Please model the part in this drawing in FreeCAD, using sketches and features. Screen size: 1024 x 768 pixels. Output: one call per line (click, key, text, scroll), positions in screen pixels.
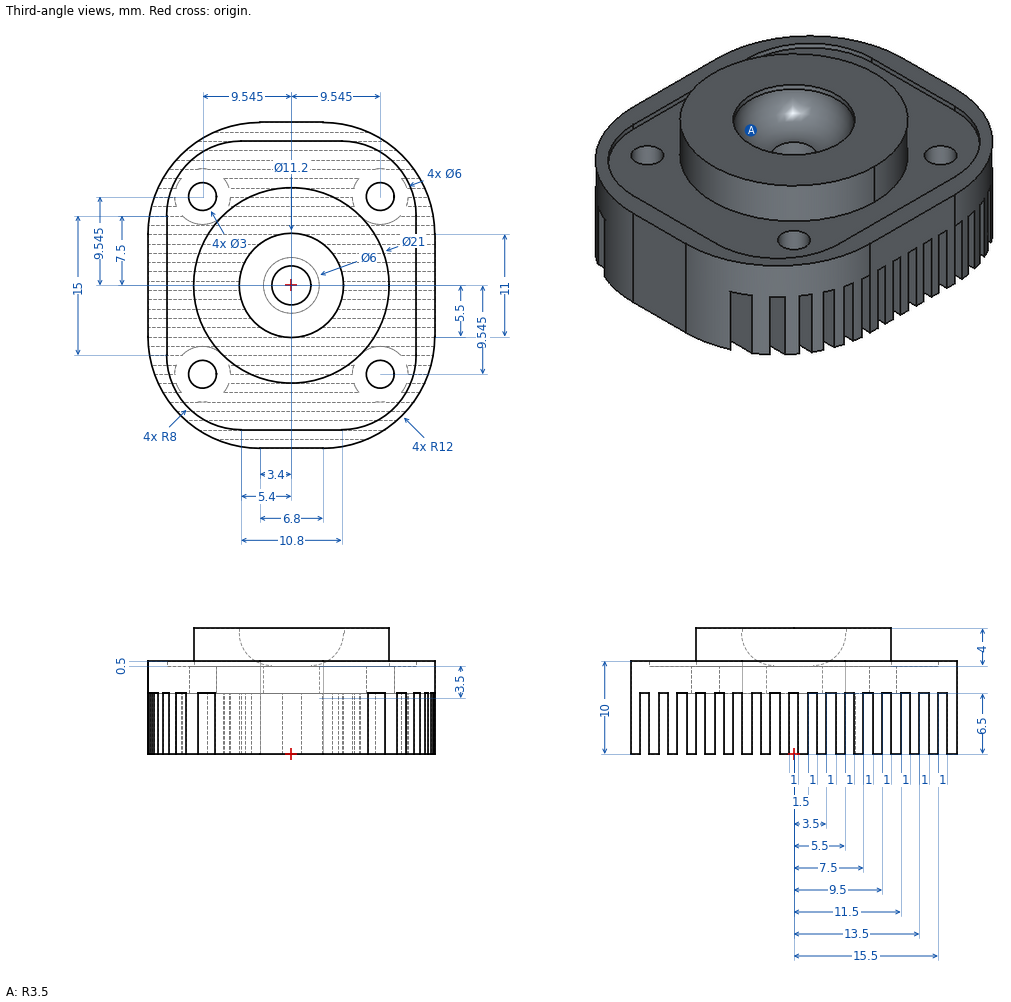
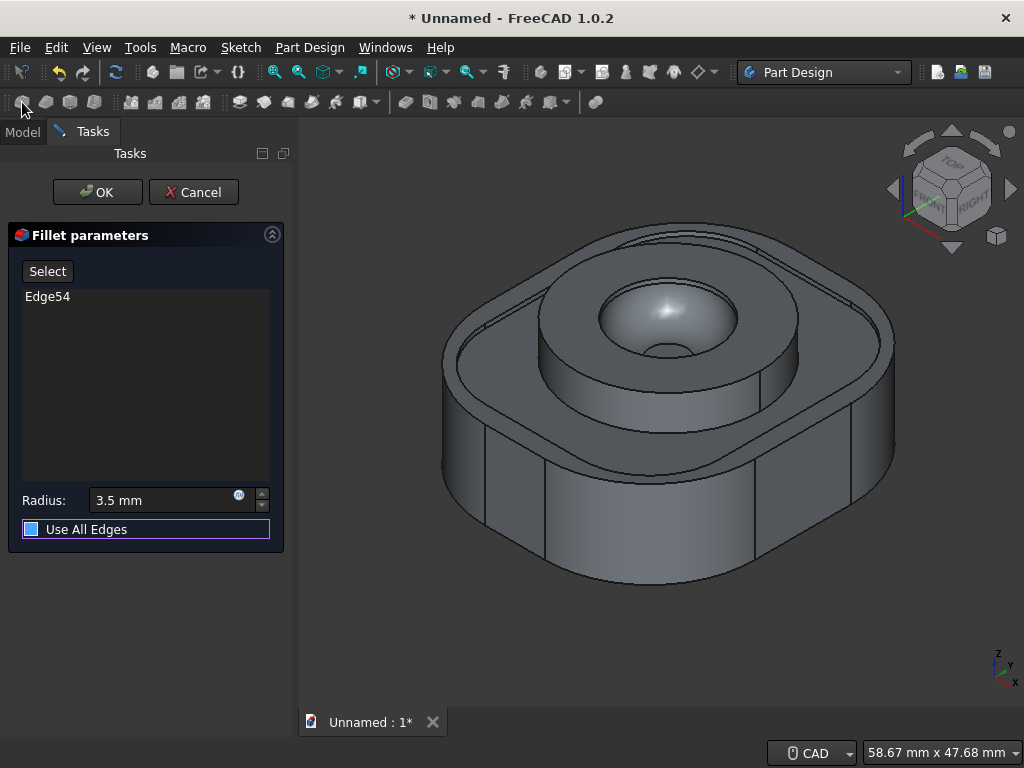
click(98, 192)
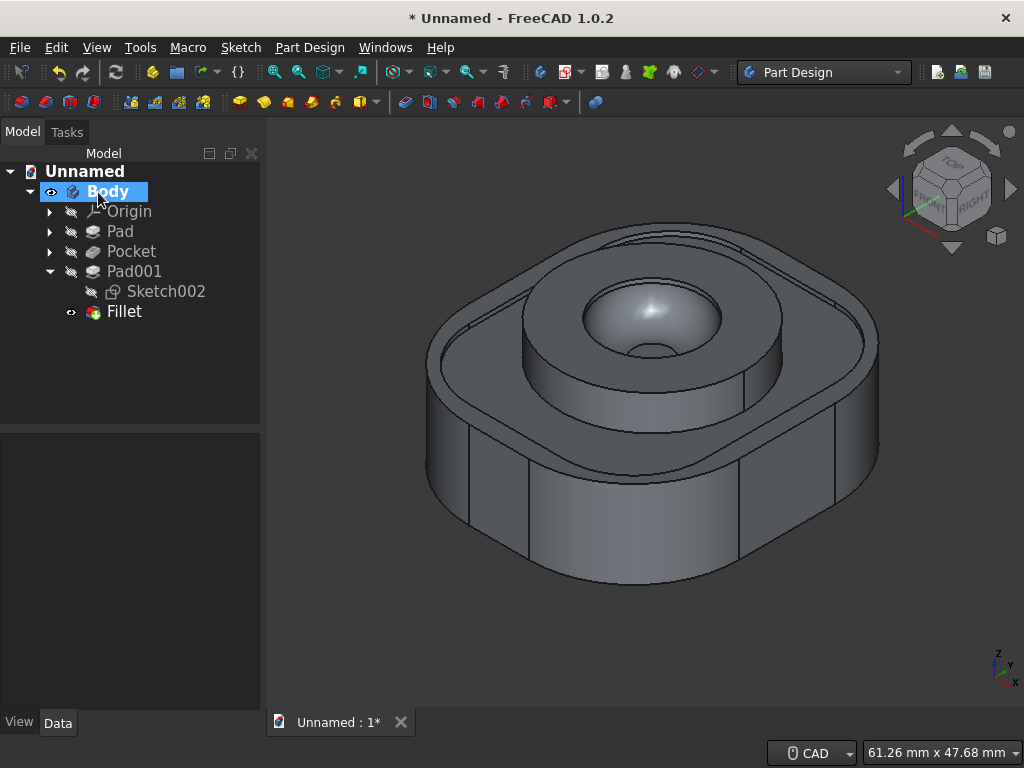
click(802, 310)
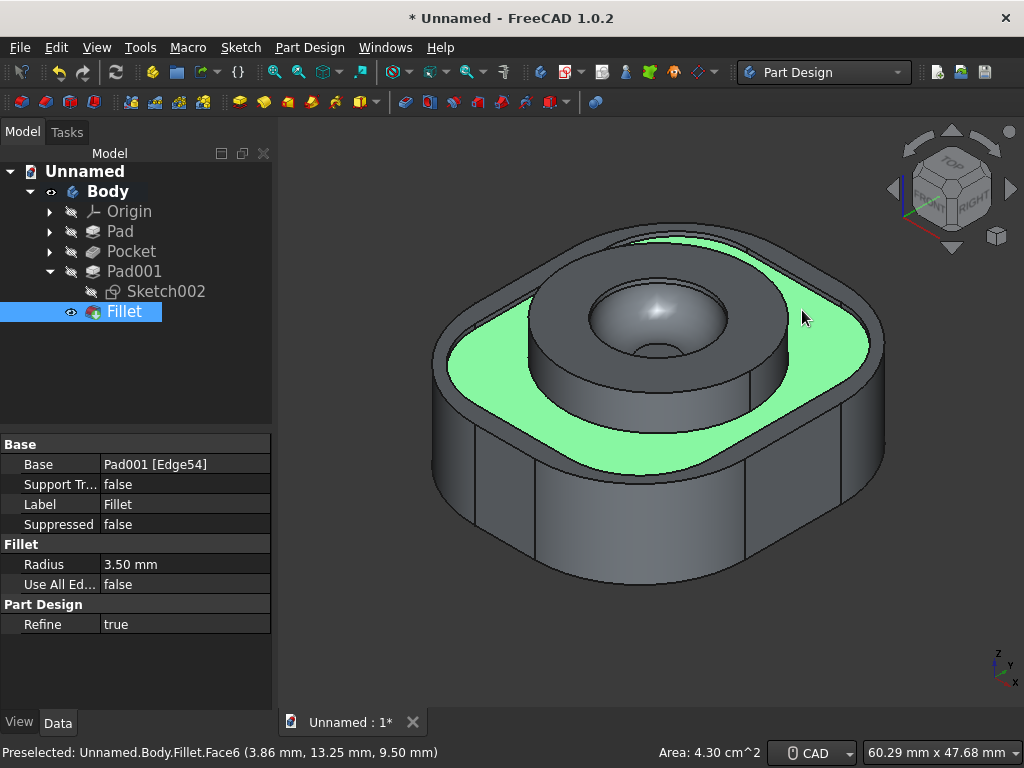
click(566, 72)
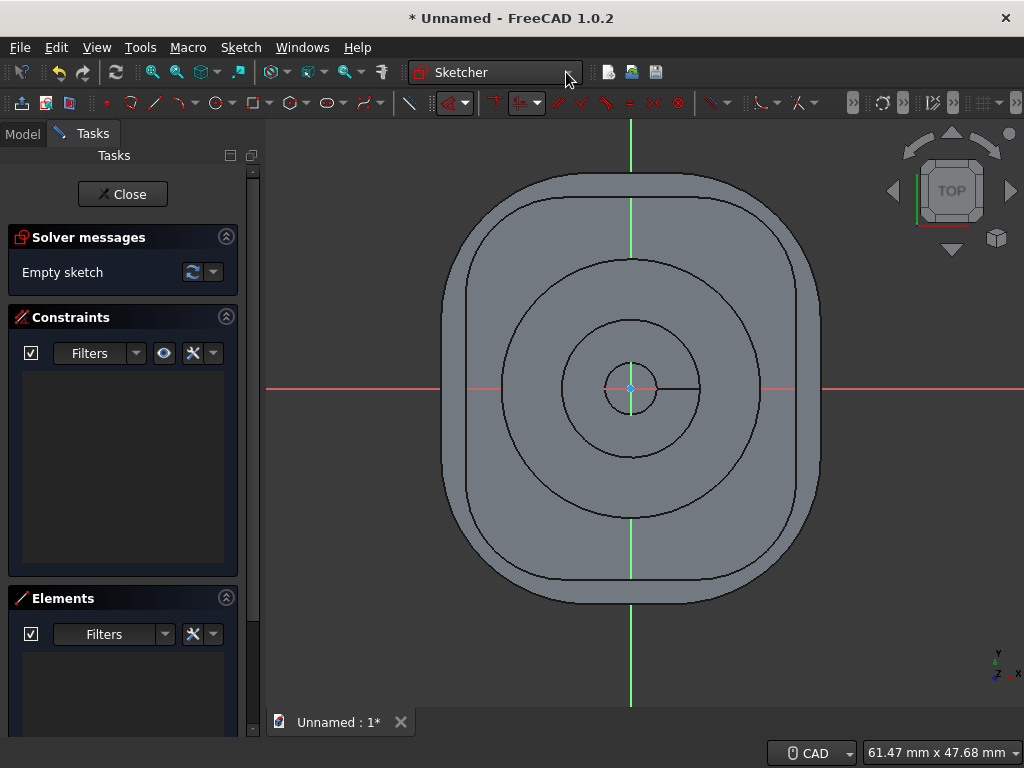
scroll(645, 382, up, 8)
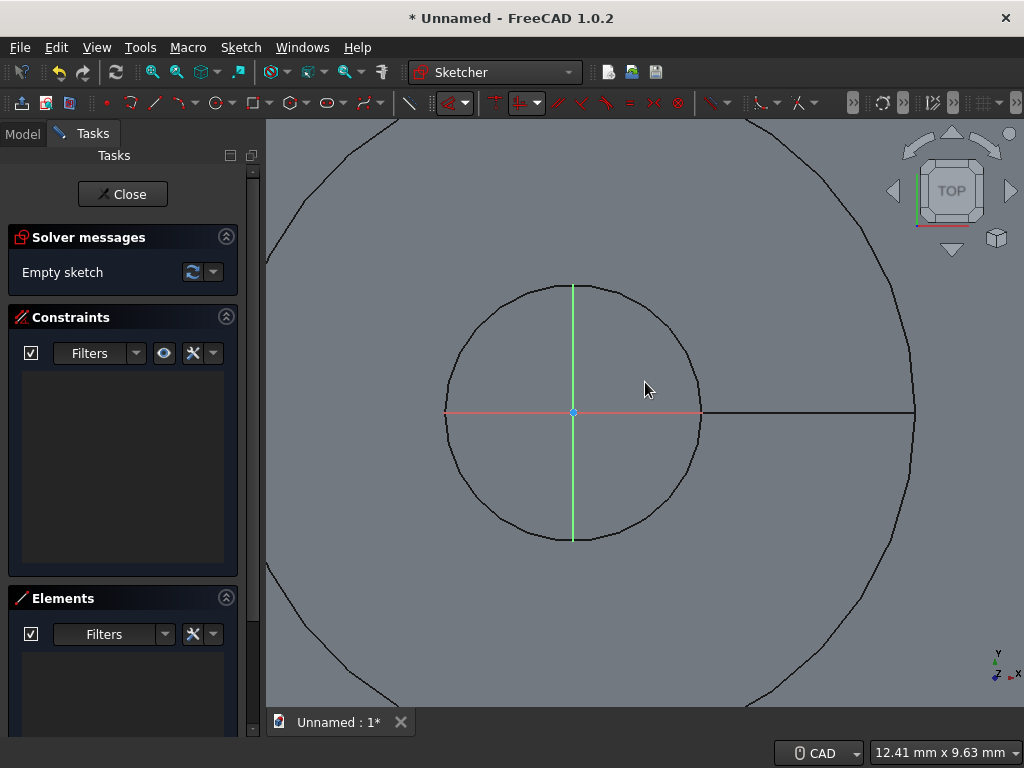
key(g)
key(c)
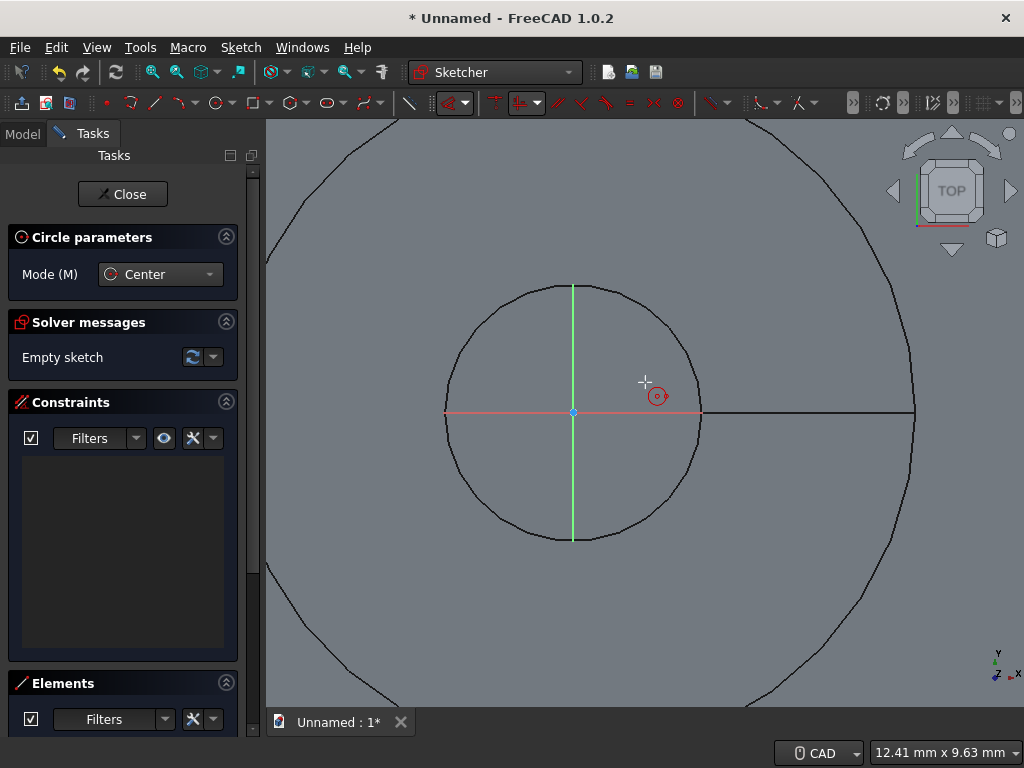
click(573, 413)
move(703, 283)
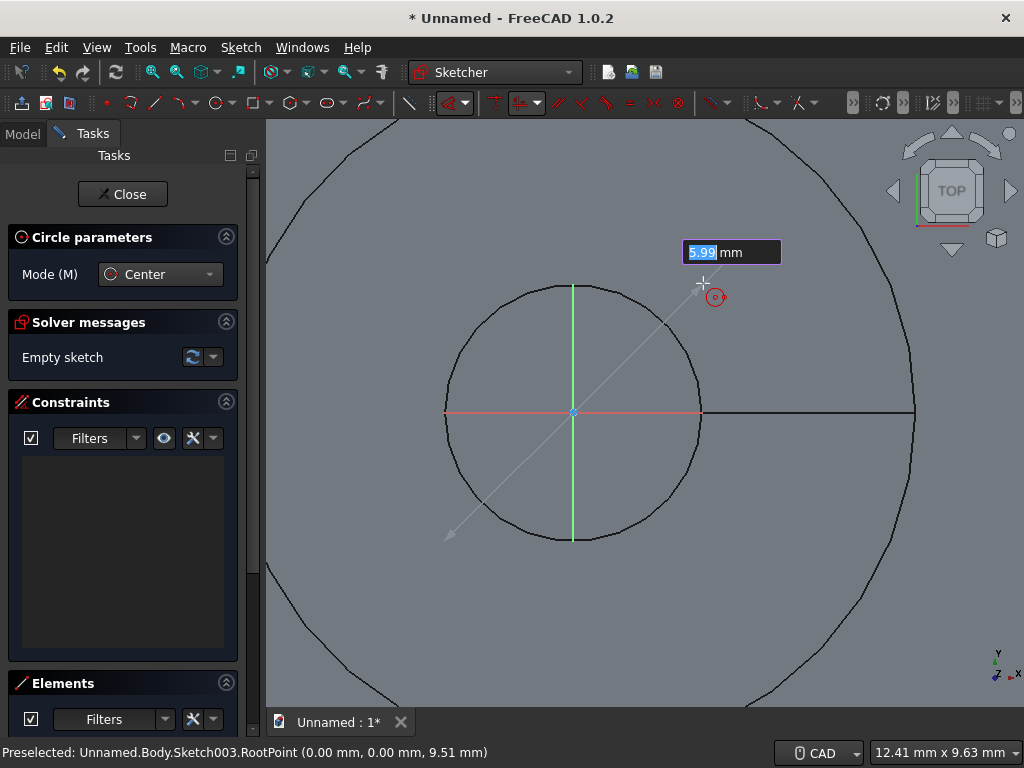
text(6)
key(Return)
key(Escape)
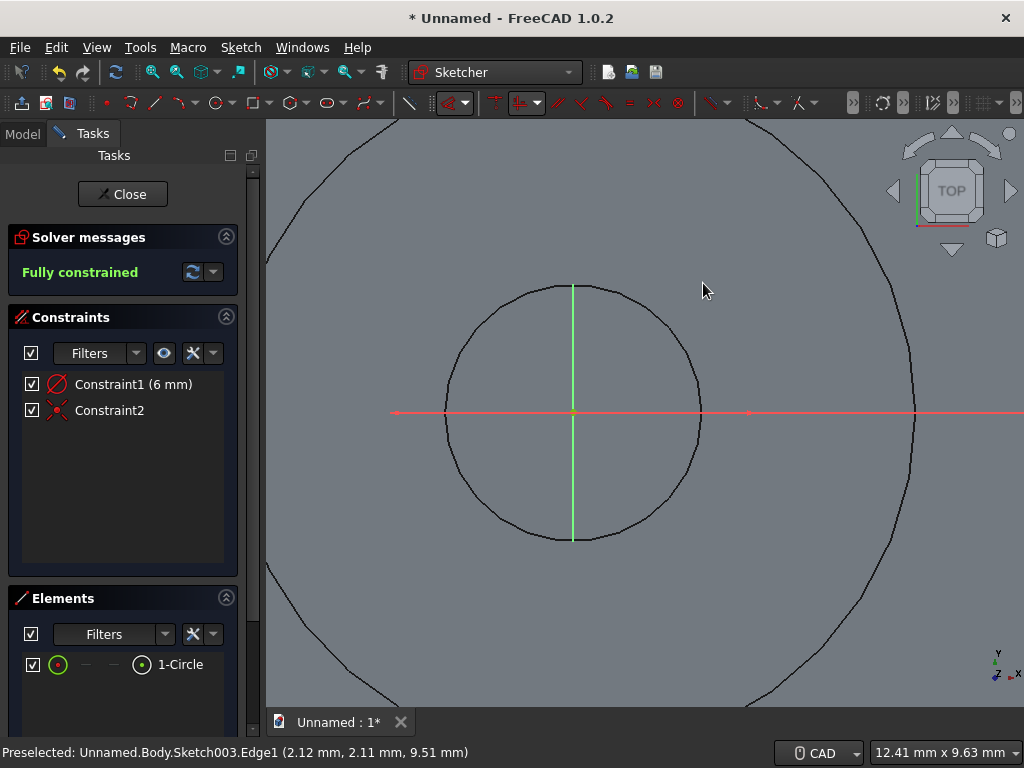
click(123, 194)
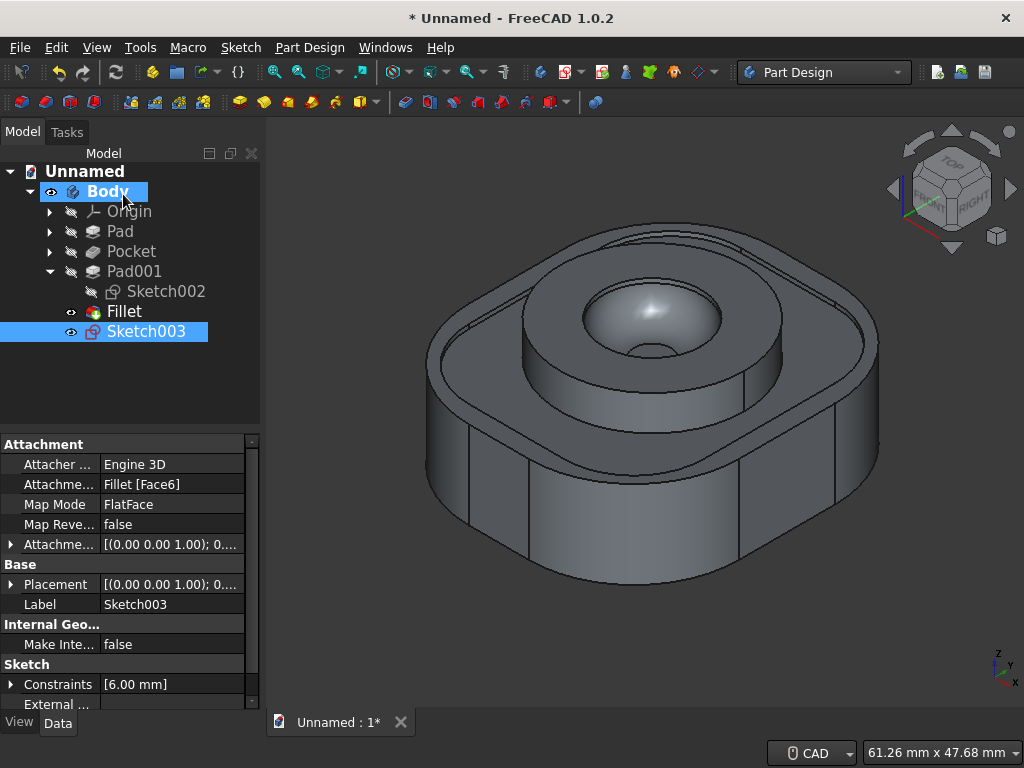
click(406, 102)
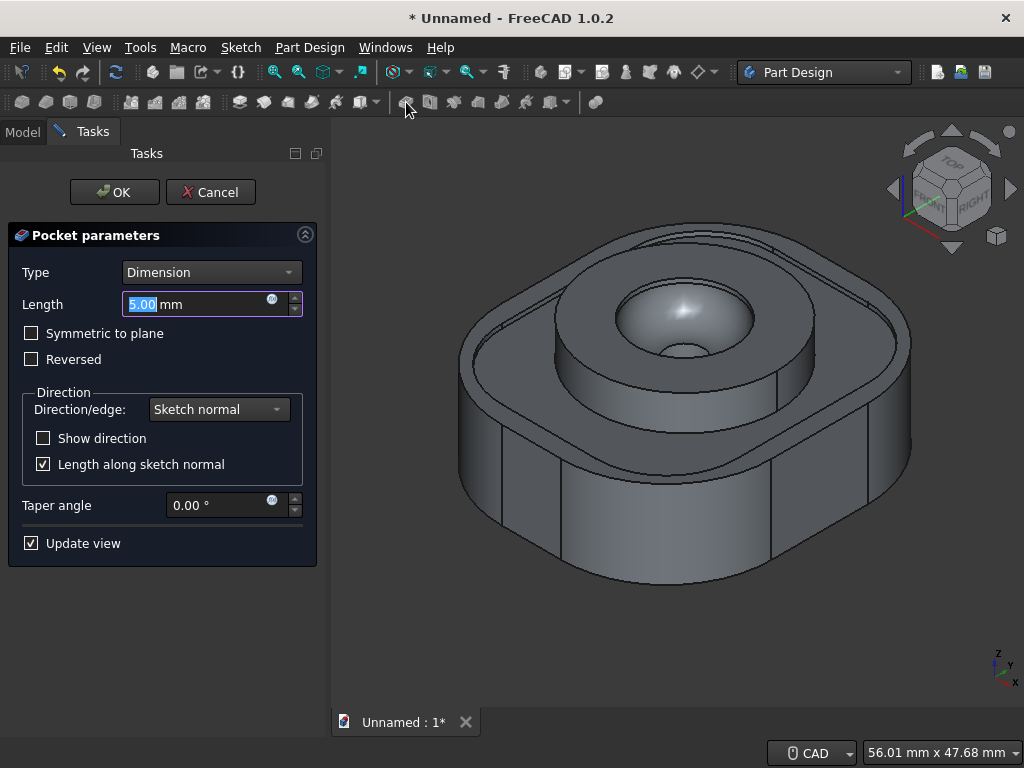
text(3.5)
key(Tab)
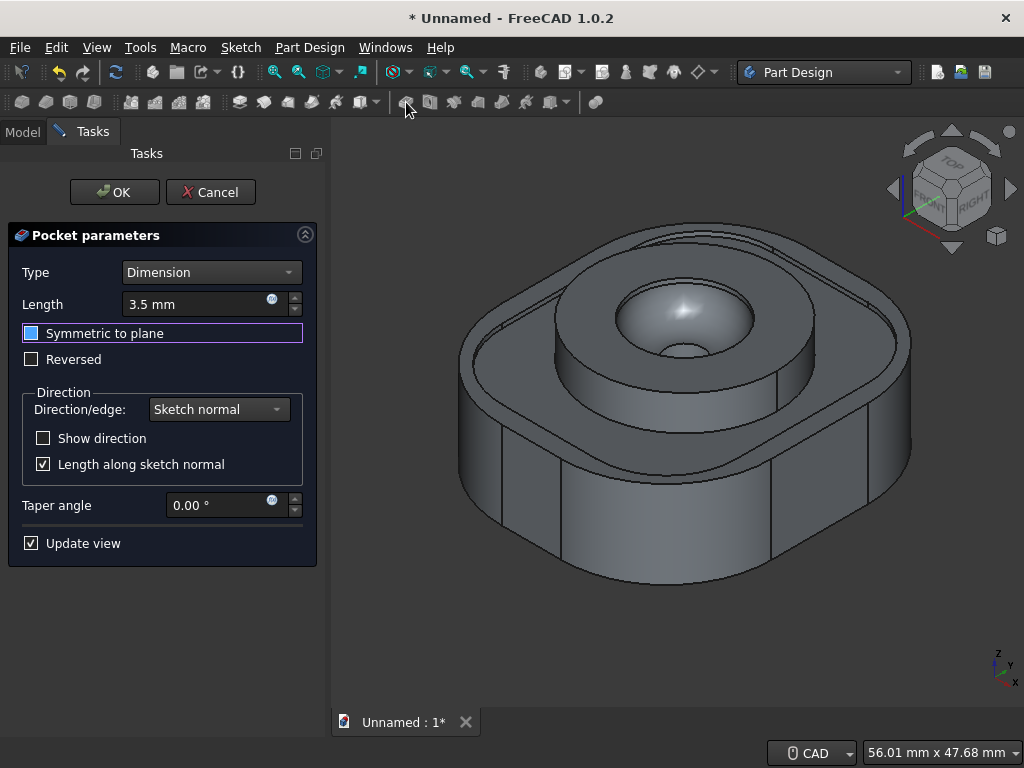
click(115, 192)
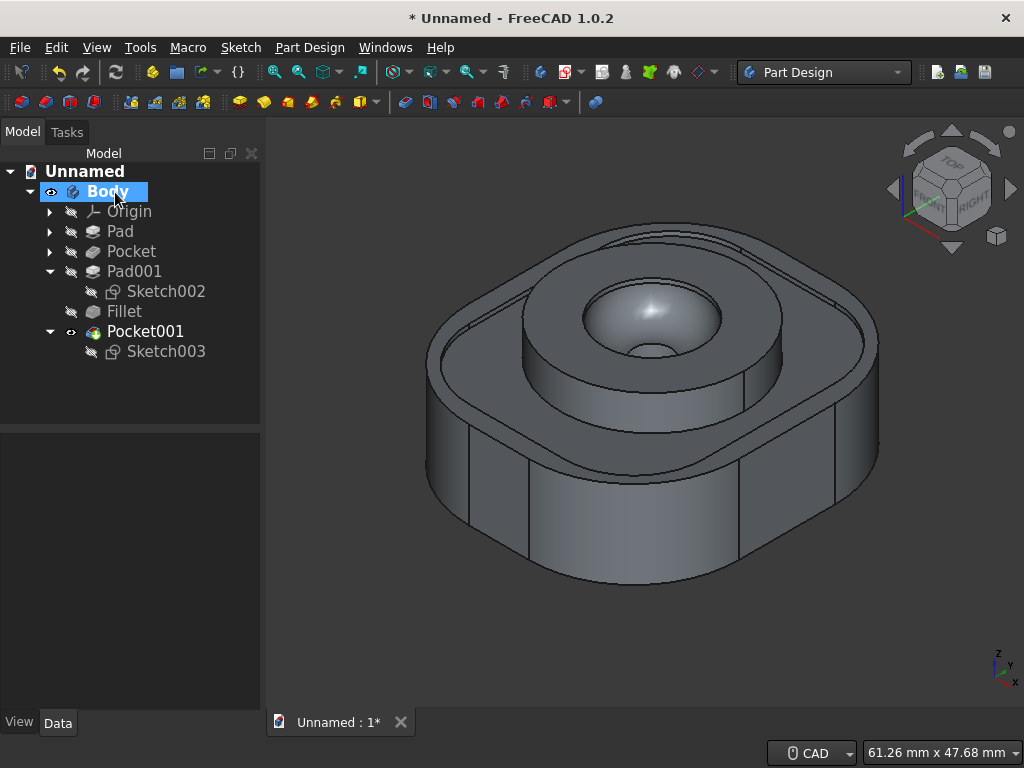
click(566, 72)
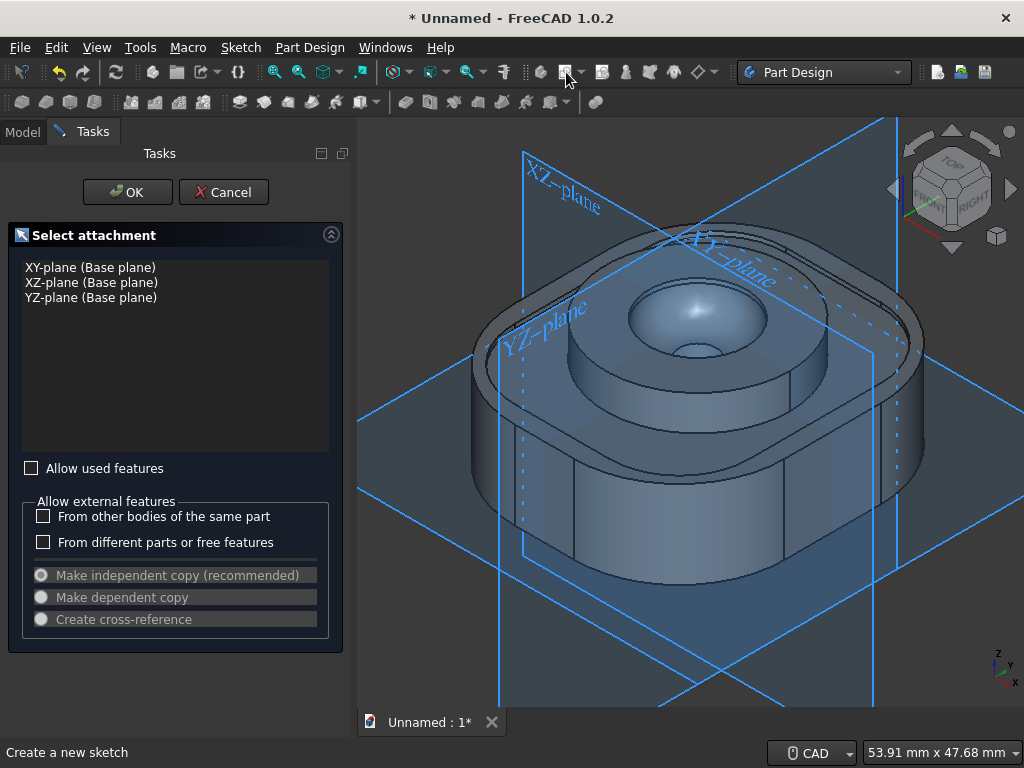
click(82, 298)